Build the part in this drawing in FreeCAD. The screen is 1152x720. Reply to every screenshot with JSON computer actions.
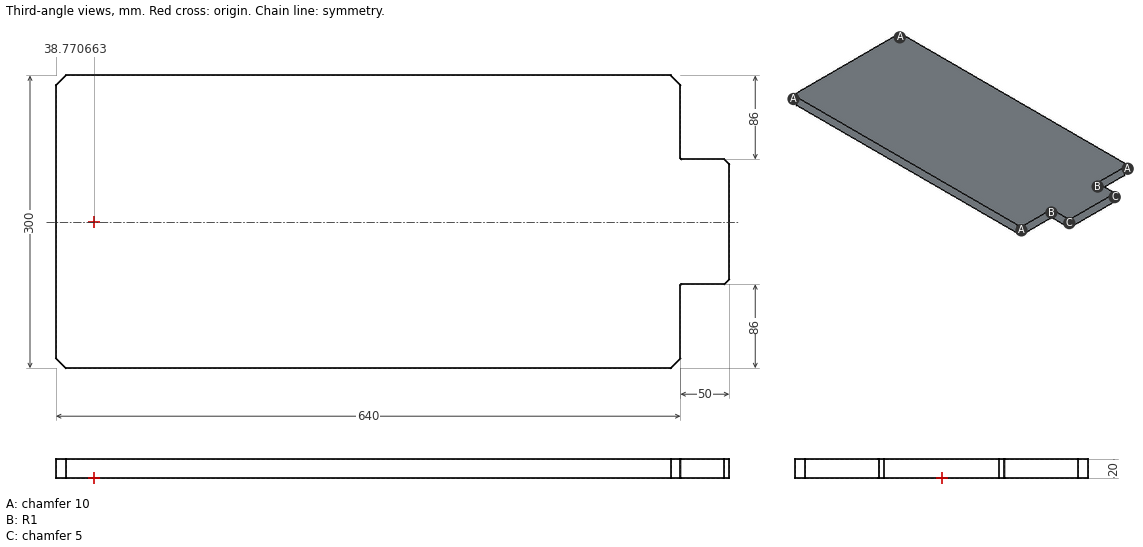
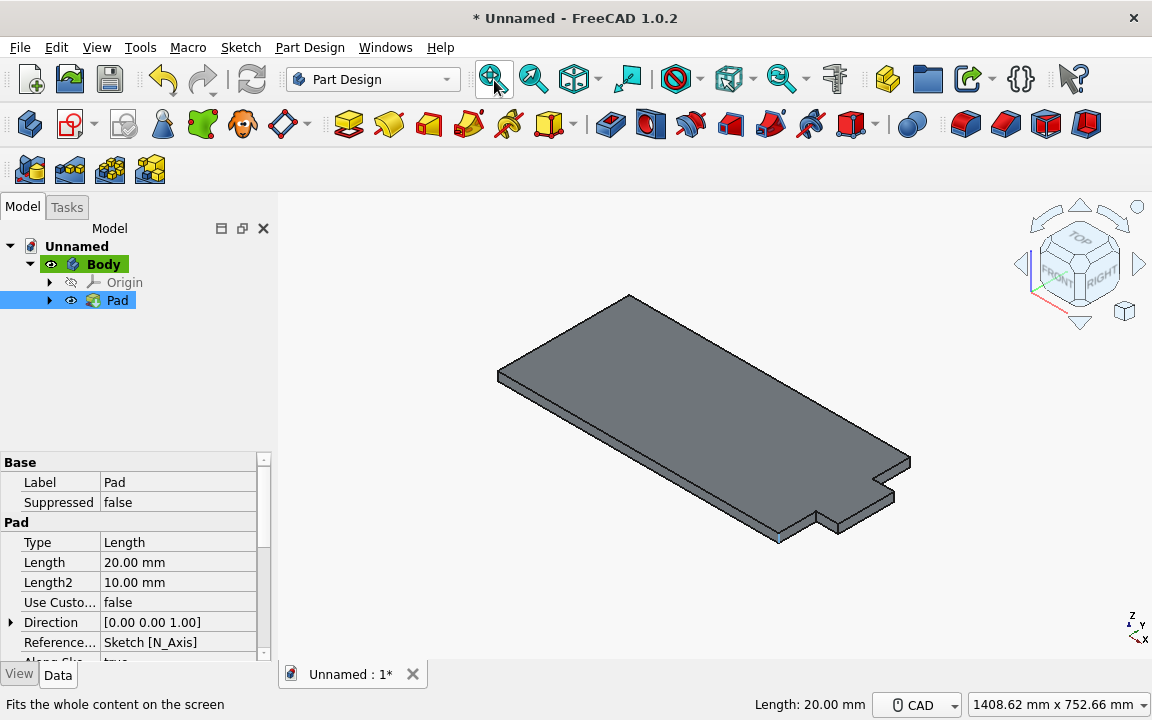
{"action": "key", "text": "2"}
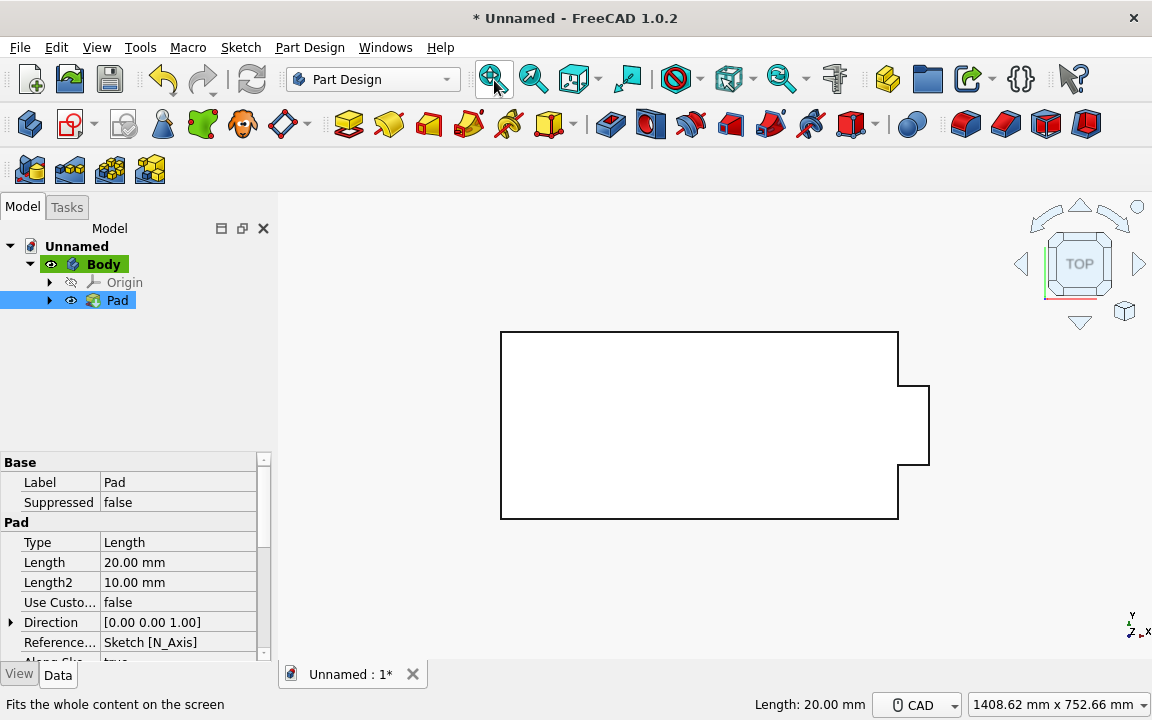
{"action": "scroll", "coordinate": [898, 331], "scroll_direction": "up", "scroll_amount": 6}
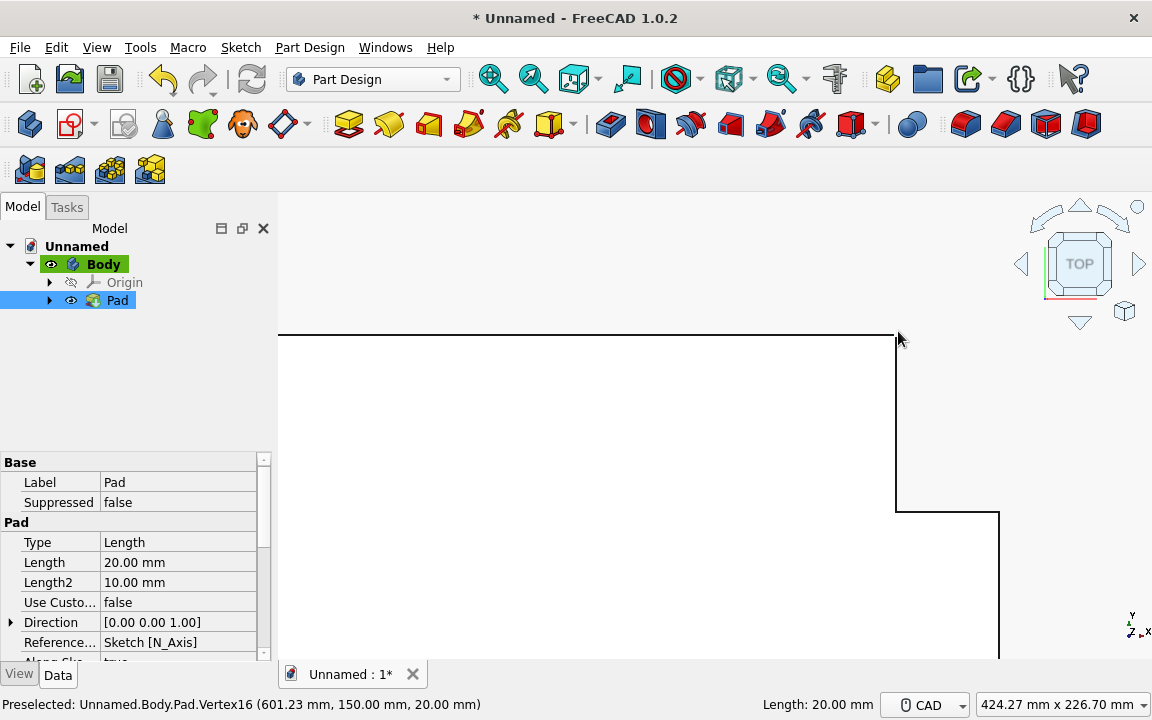
{"action": "left_click", "coordinate": [494, 80]}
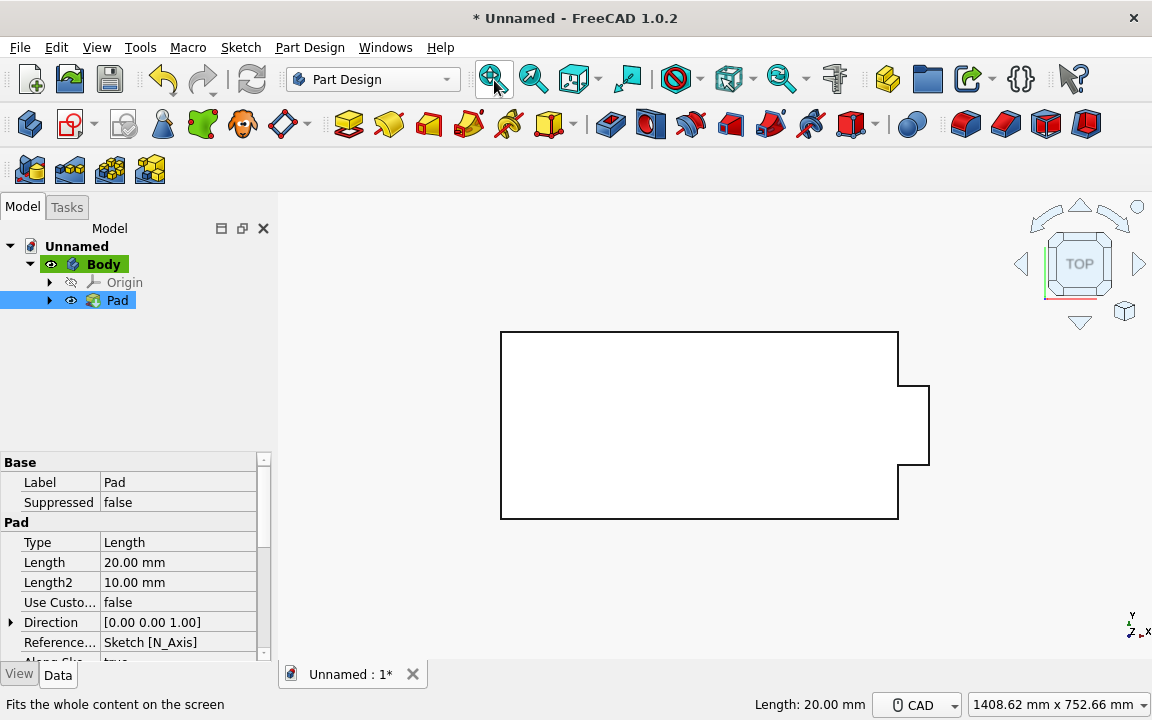
{"action": "key", "text": "1"}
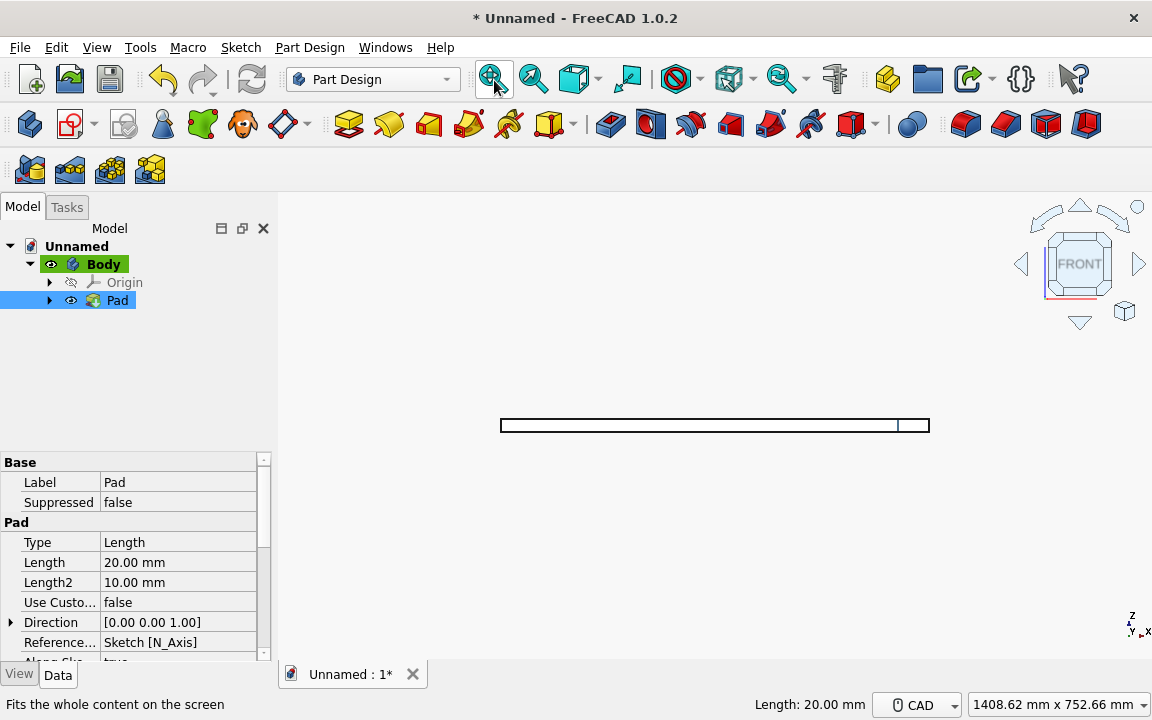
{"action": "scroll", "coordinate": [898, 424], "scroll_direction": "up", "scroll_amount": 6}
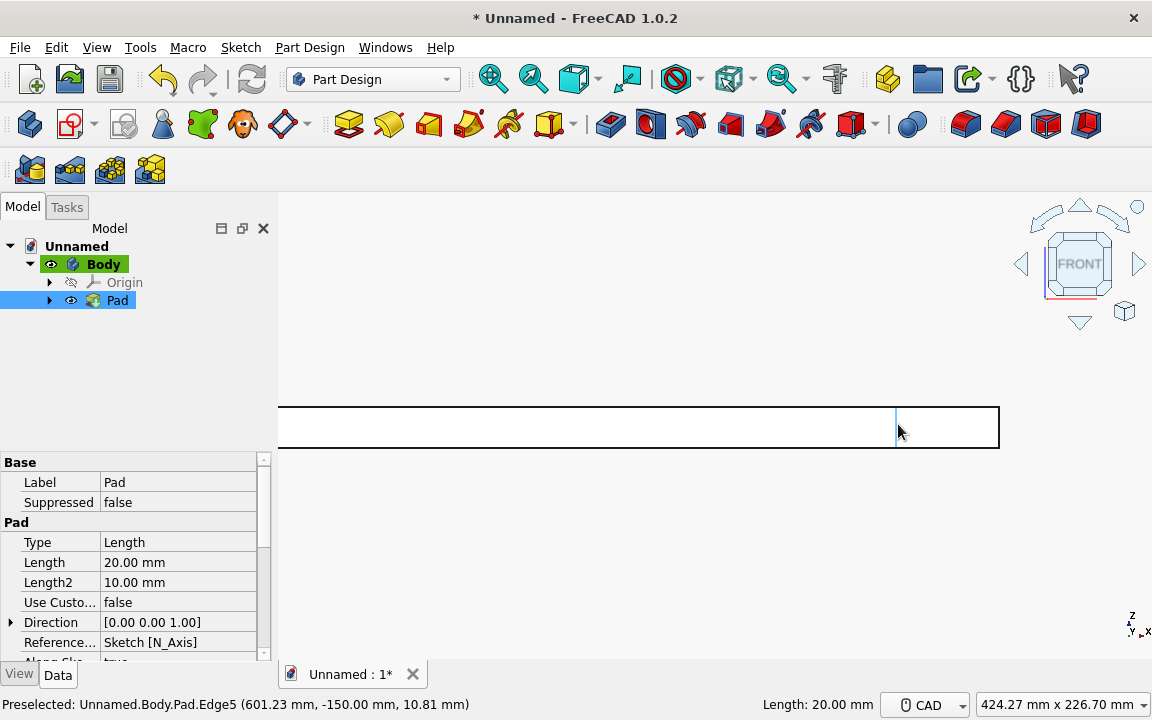
{"action": "key", "text": "v f"}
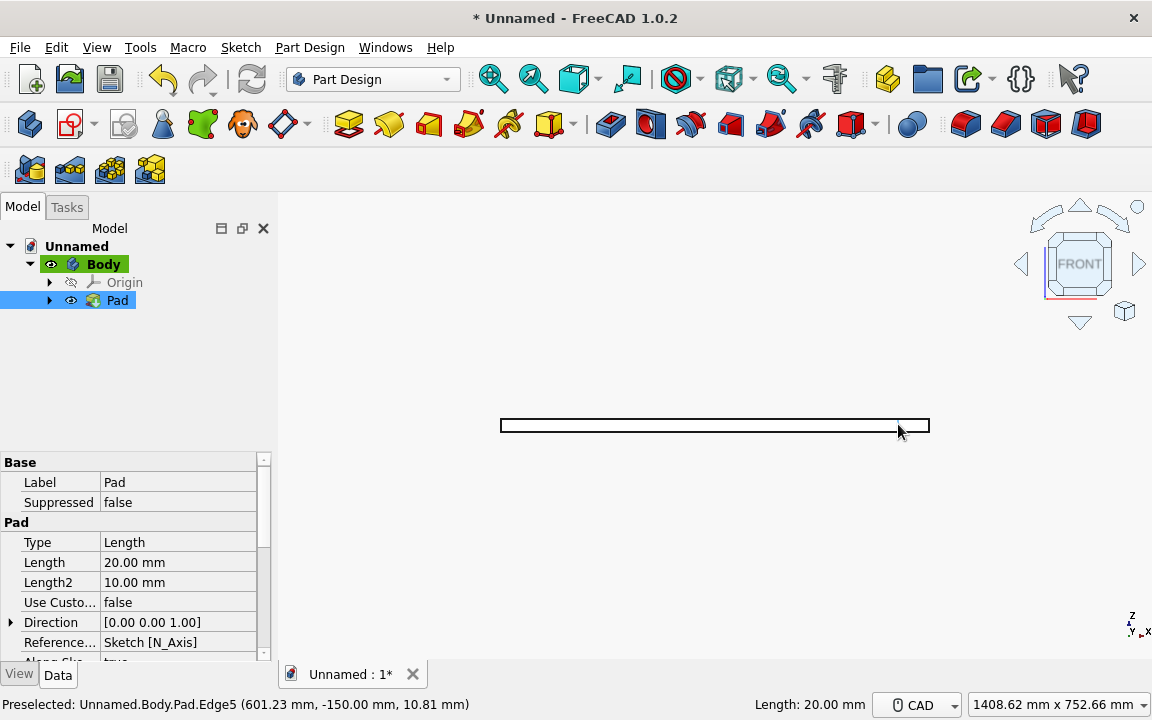
{"action": "key", "text": "3"}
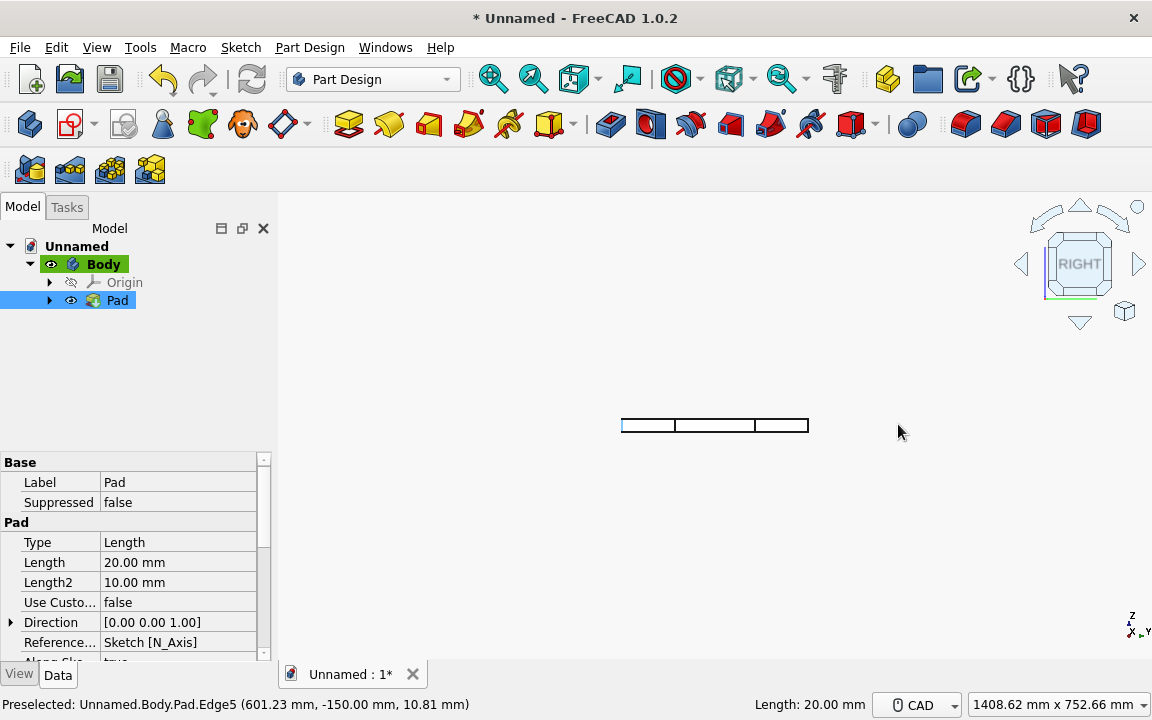
{"action": "left_click", "coordinate": [494, 80]}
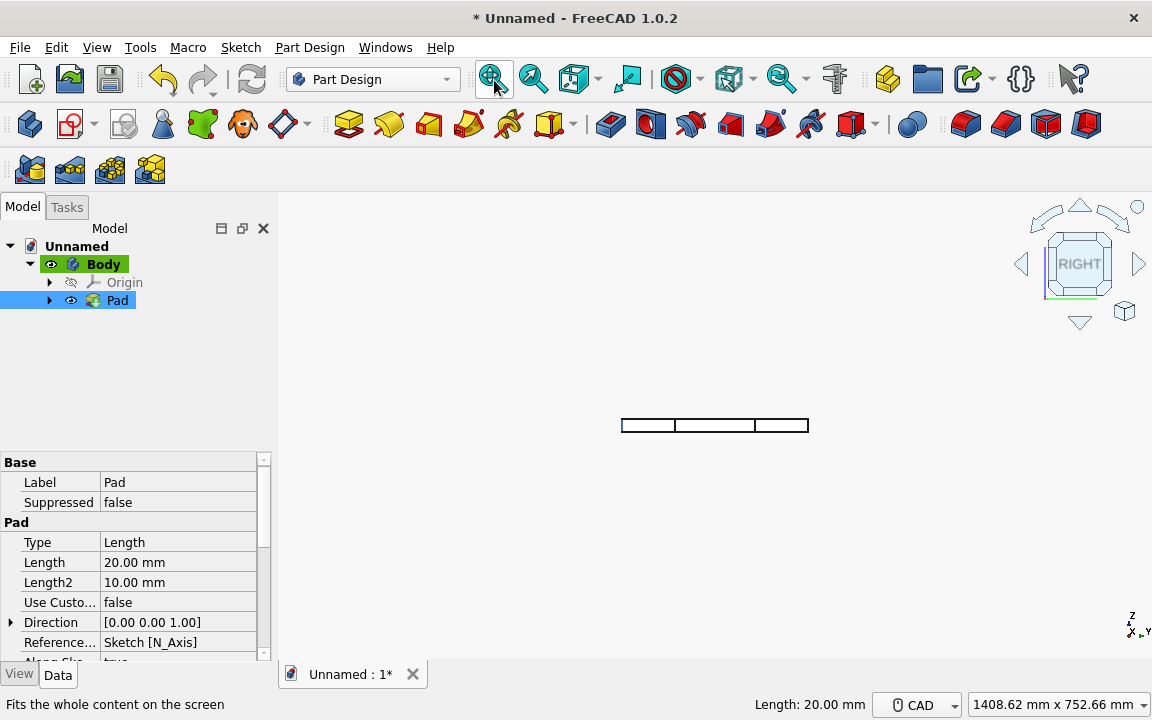
{"action": "scroll", "coordinate": [808, 424], "scroll_direction": "up", "scroll_amount": 6}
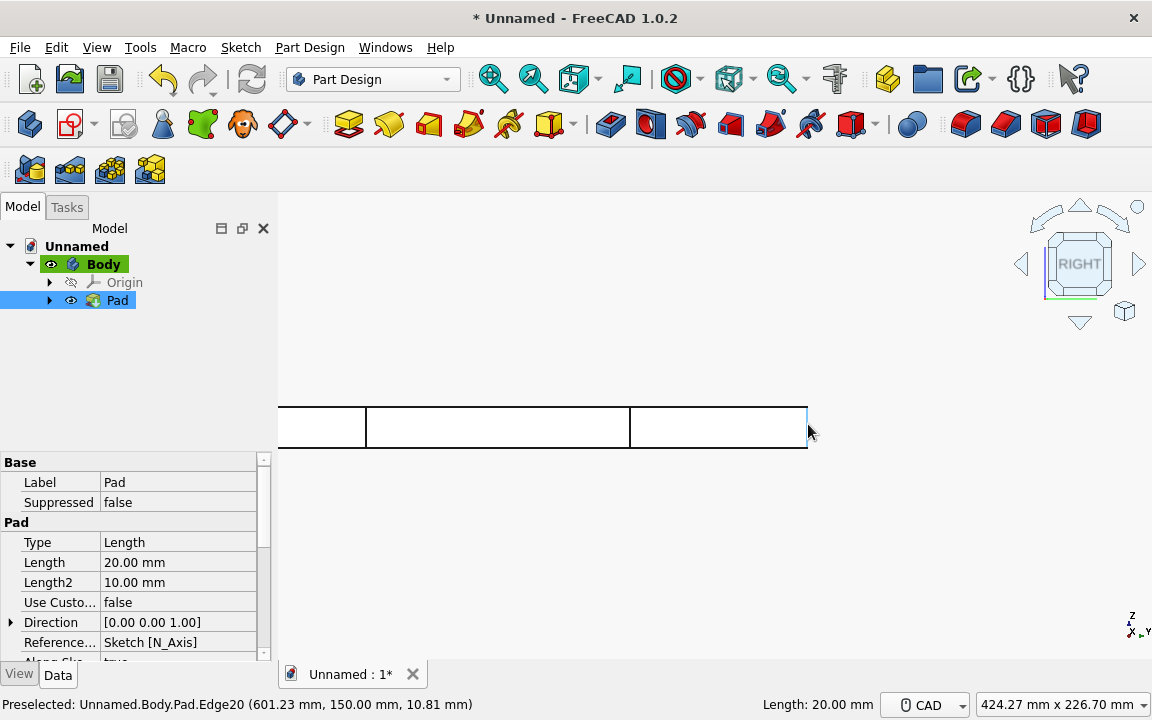
{"action": "left_click", "coordinate": [807, 427], "text": "ctrl"}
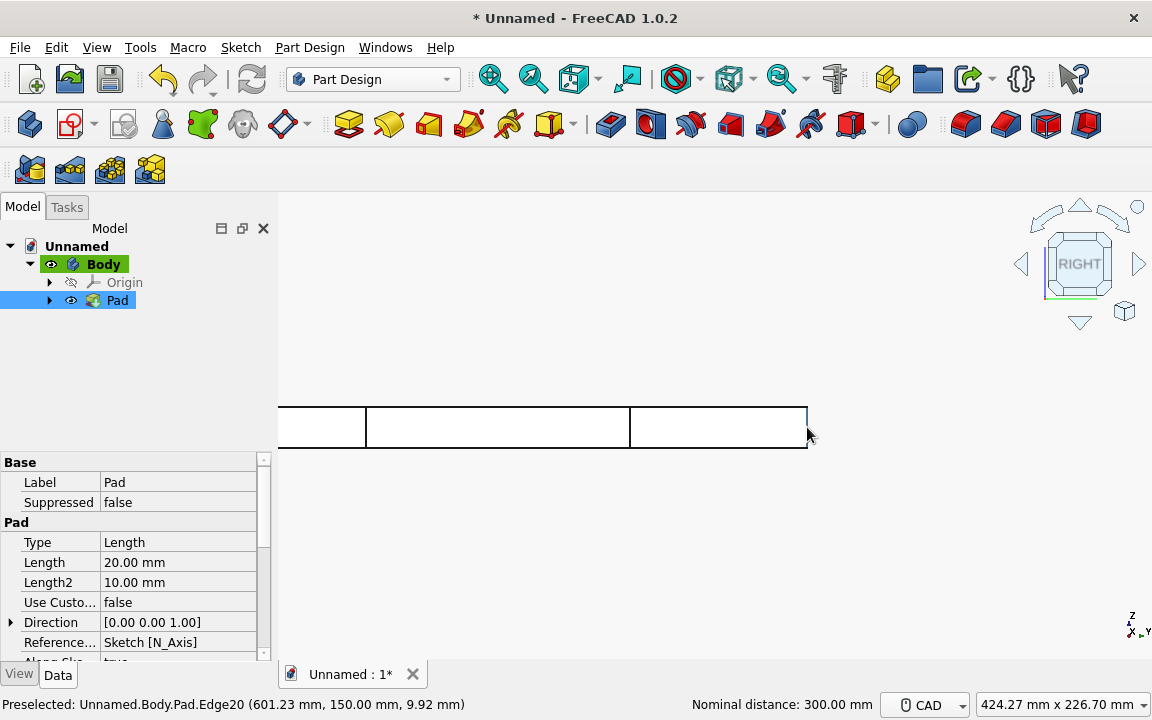
{"action": "left_click", "coordinate": [494, 80]}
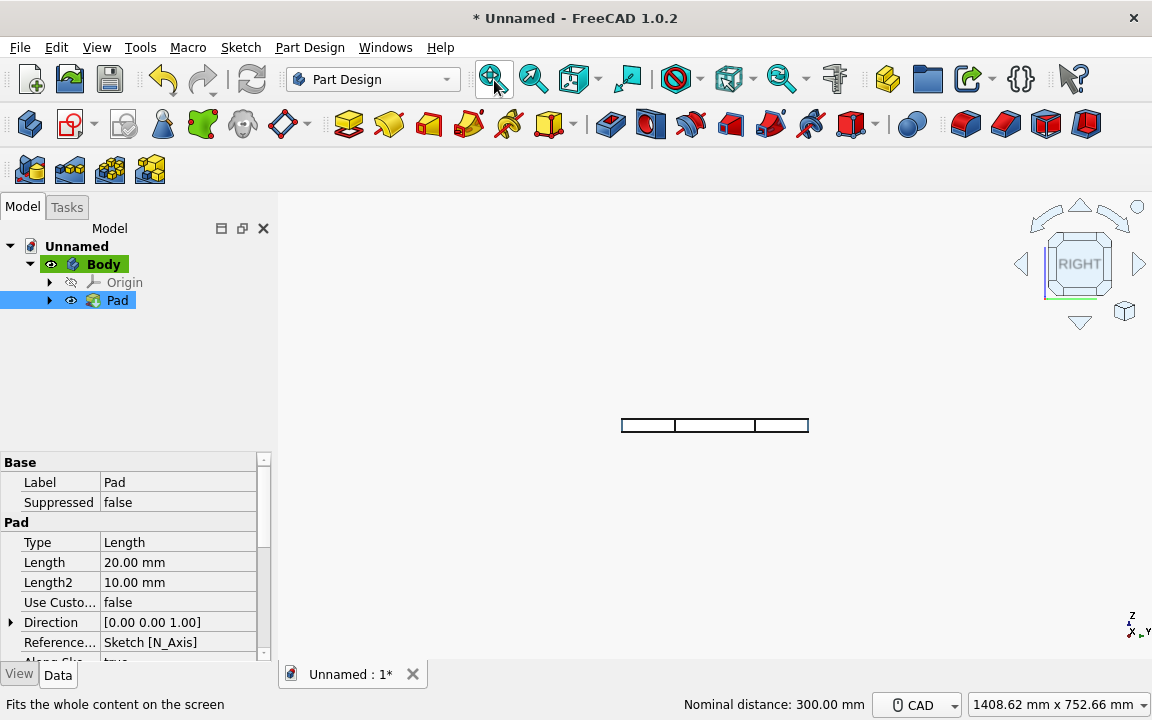
{"action": "key", "text": "5"}